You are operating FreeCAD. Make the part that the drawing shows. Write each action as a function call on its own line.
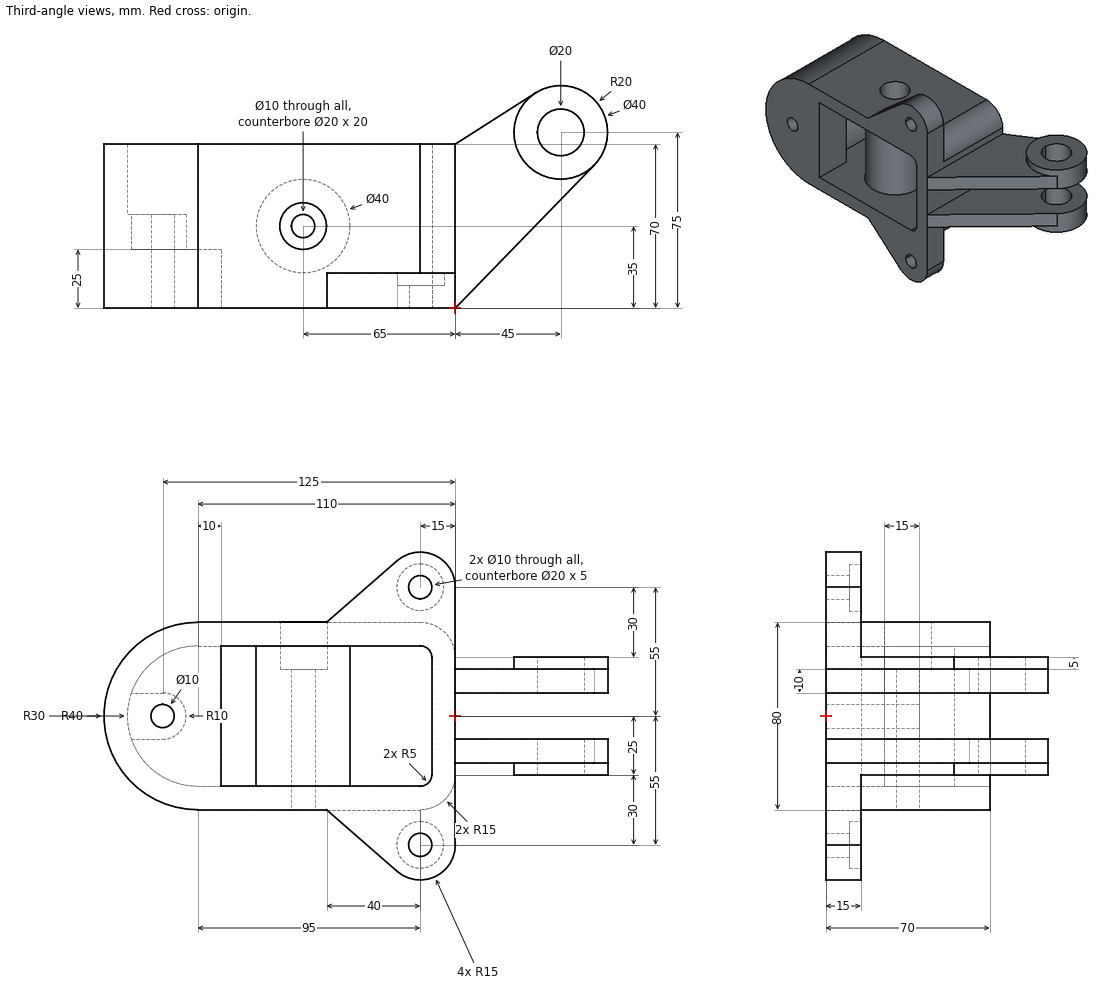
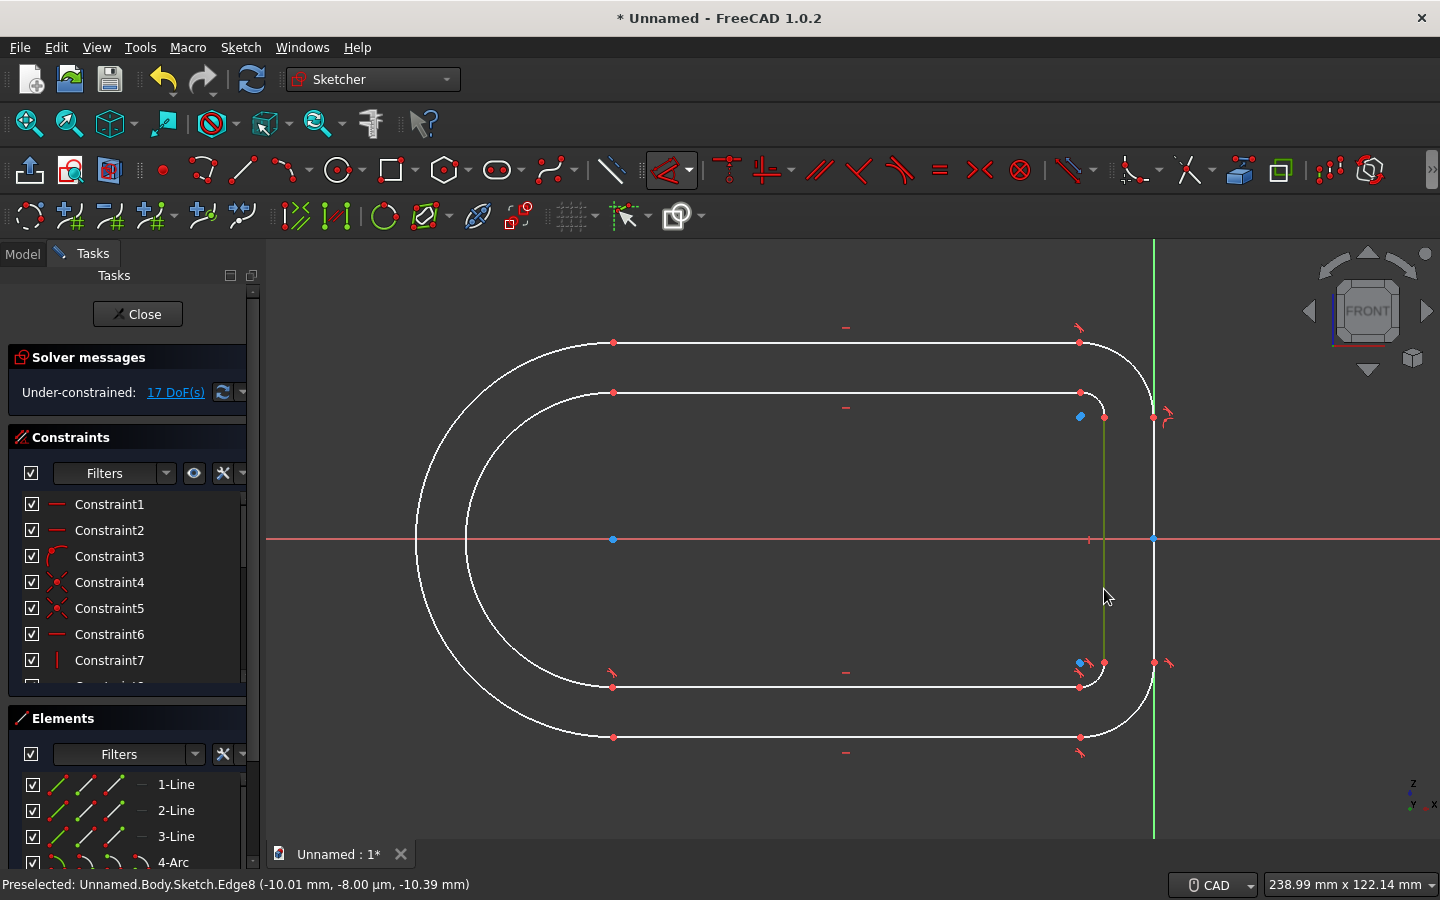
click(1102, 406)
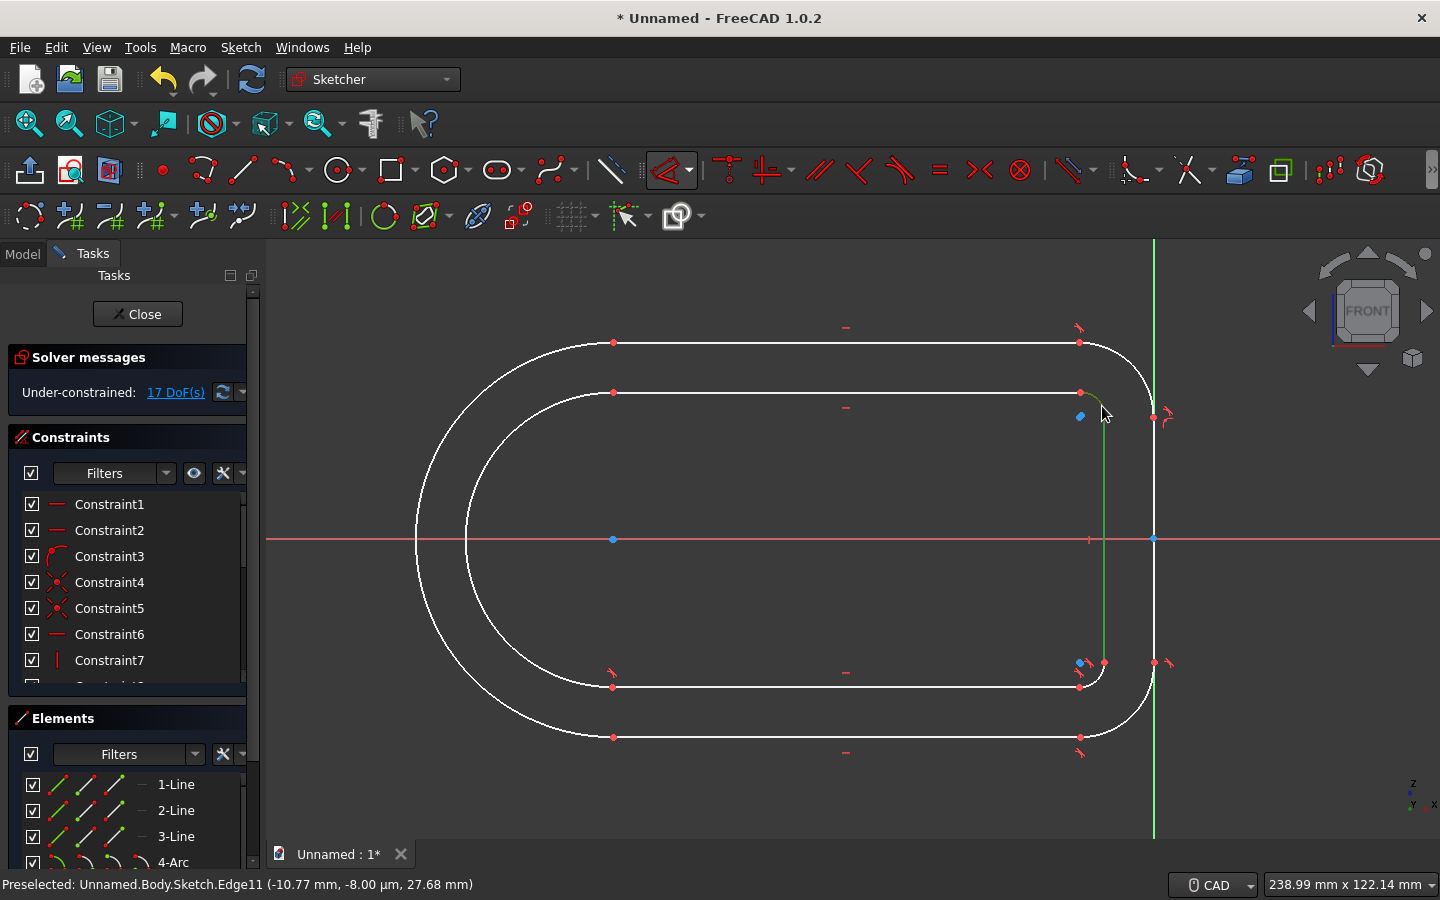
key(t)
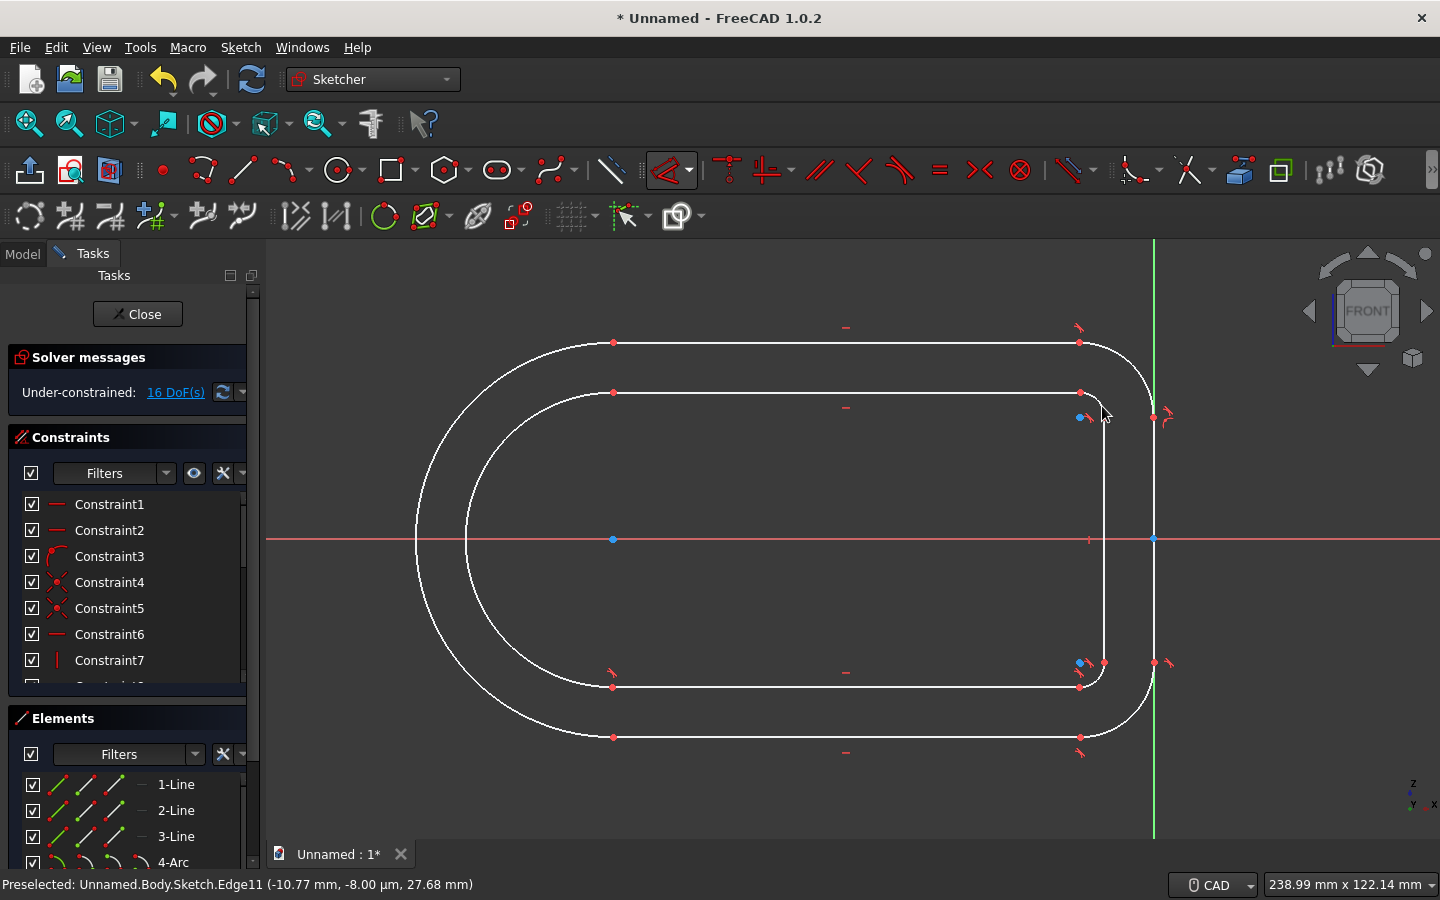
click(940, 393)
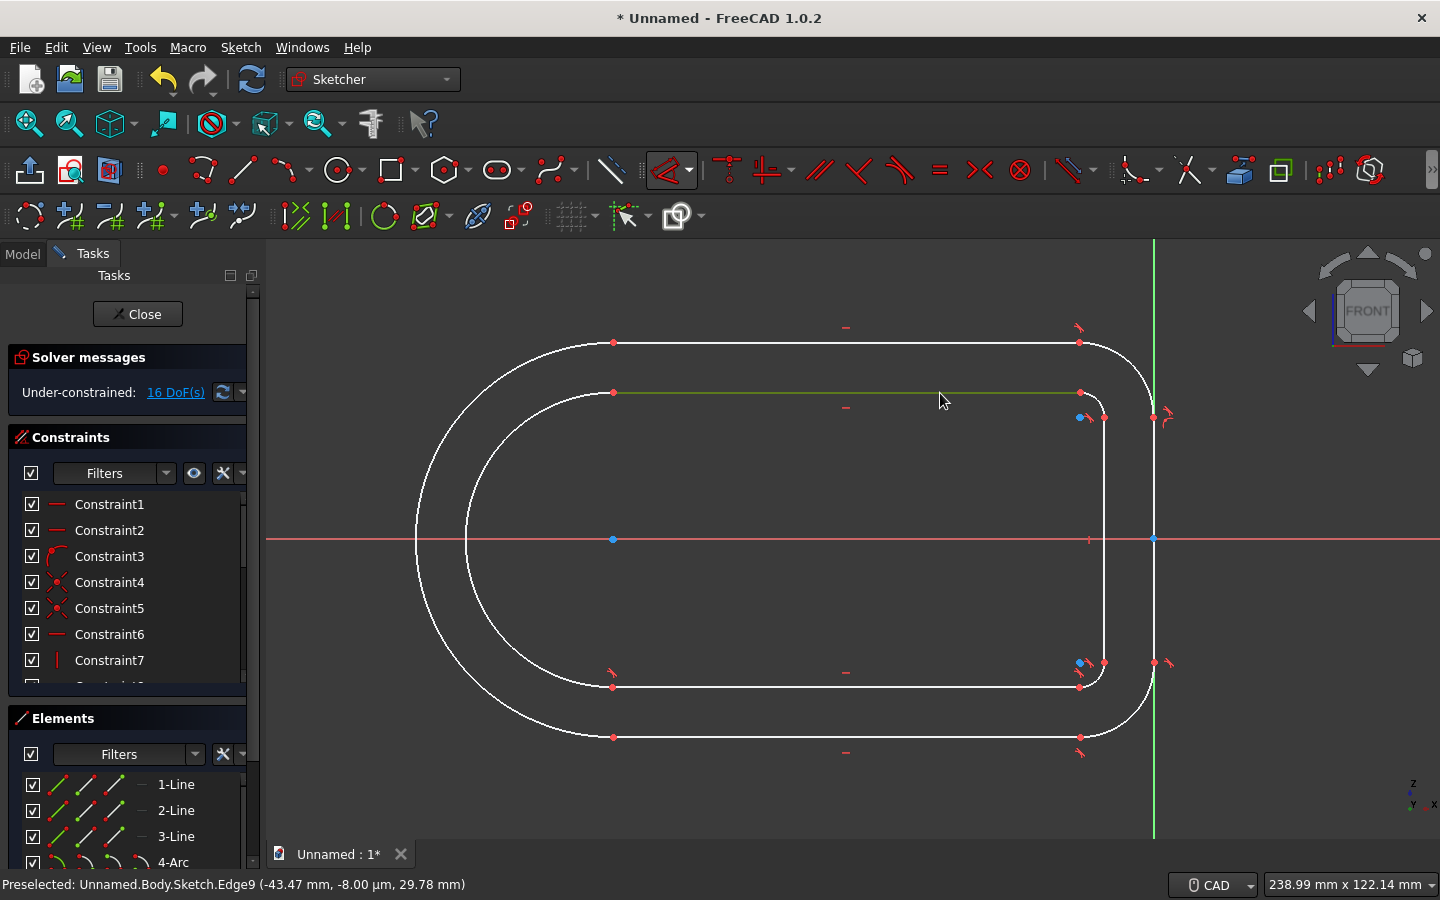
click(1102, 406)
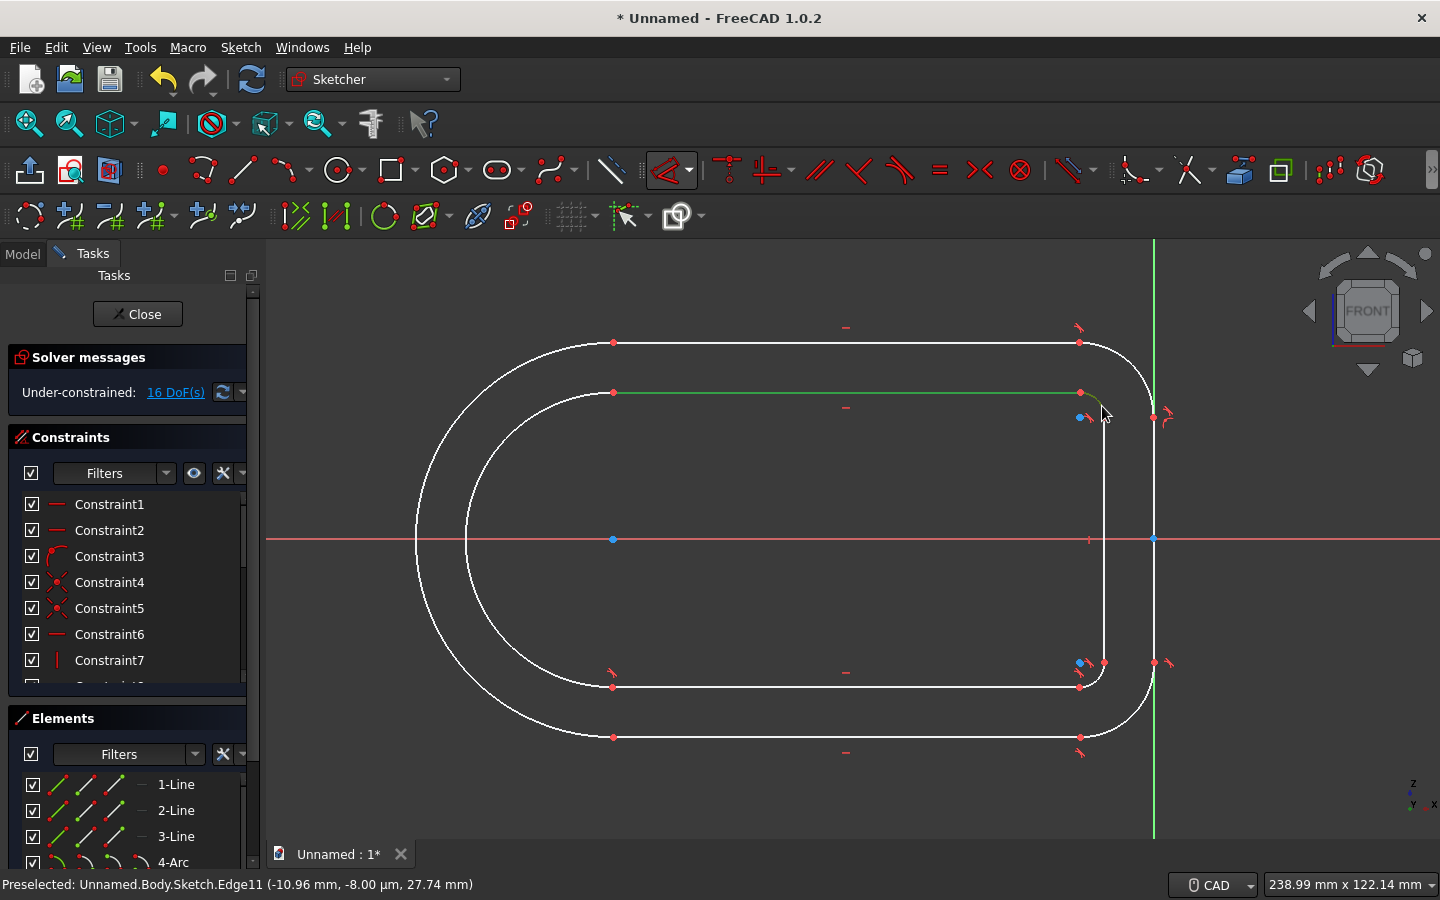
key(t)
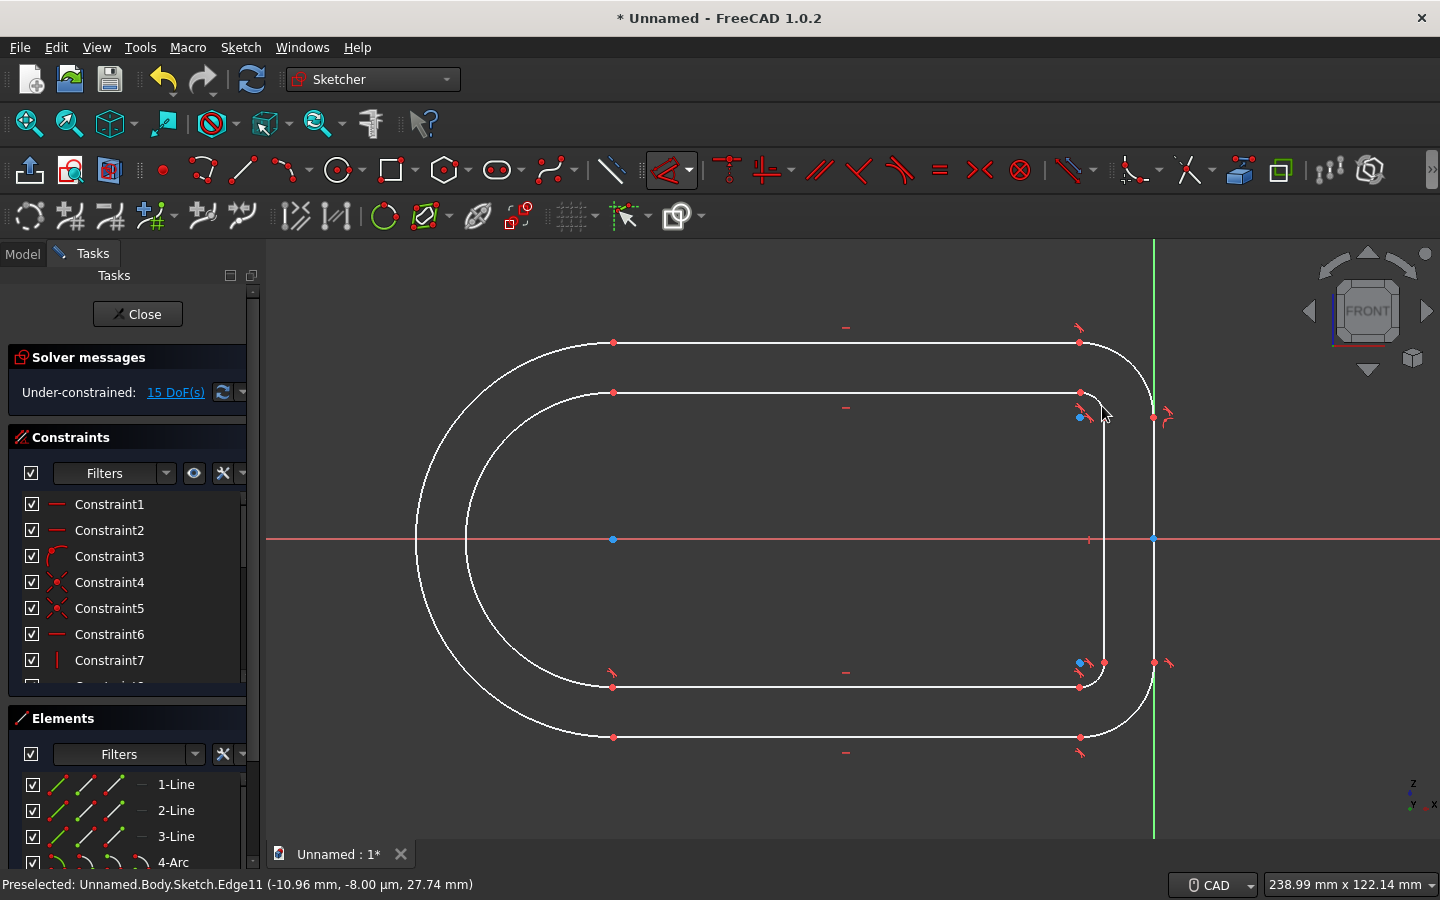
click(940, 393)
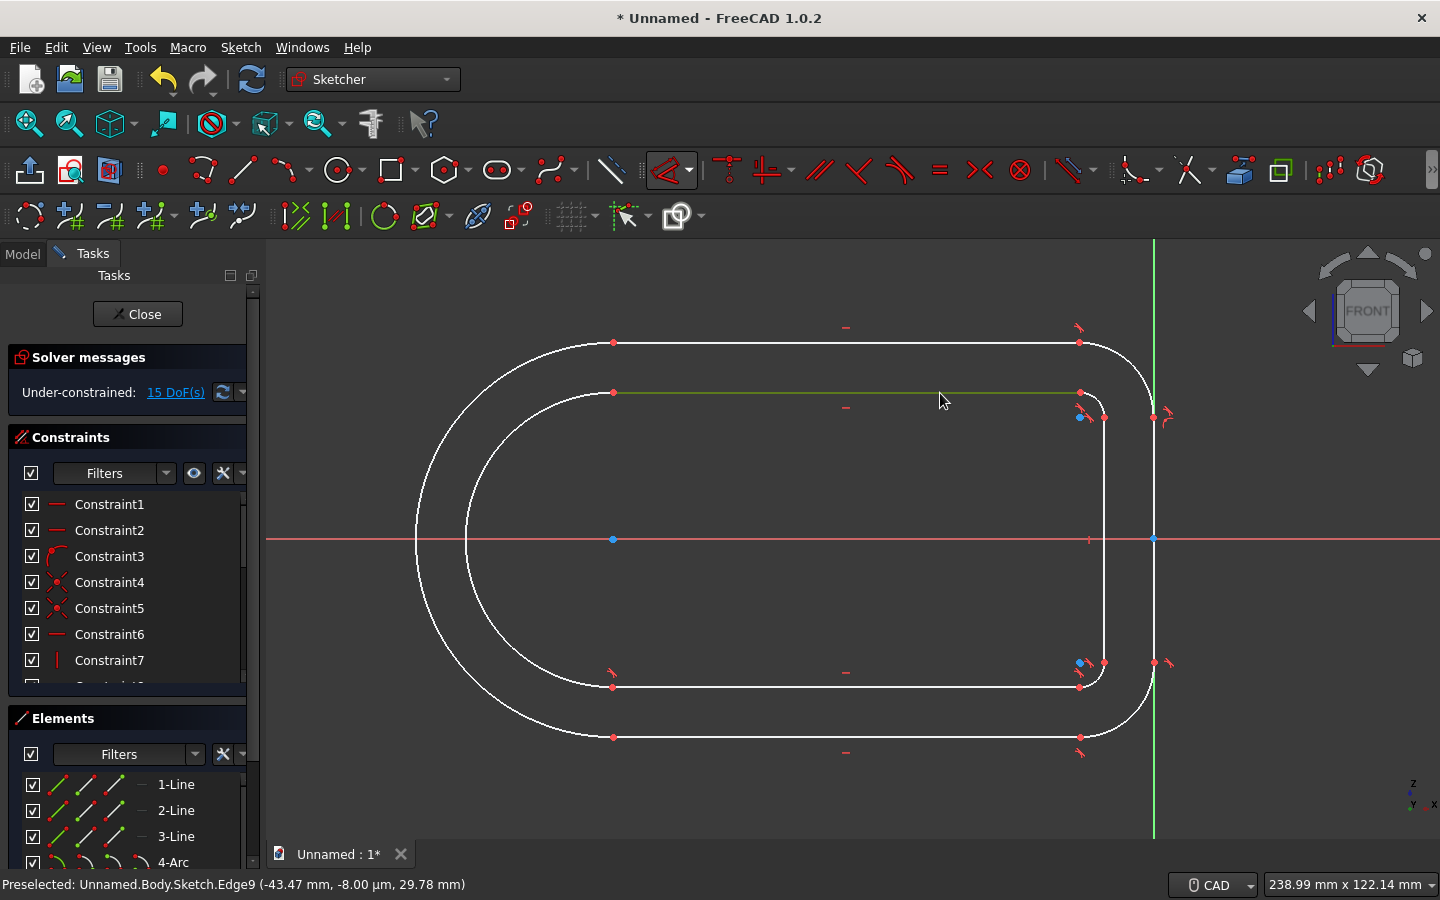
click(494, 453)